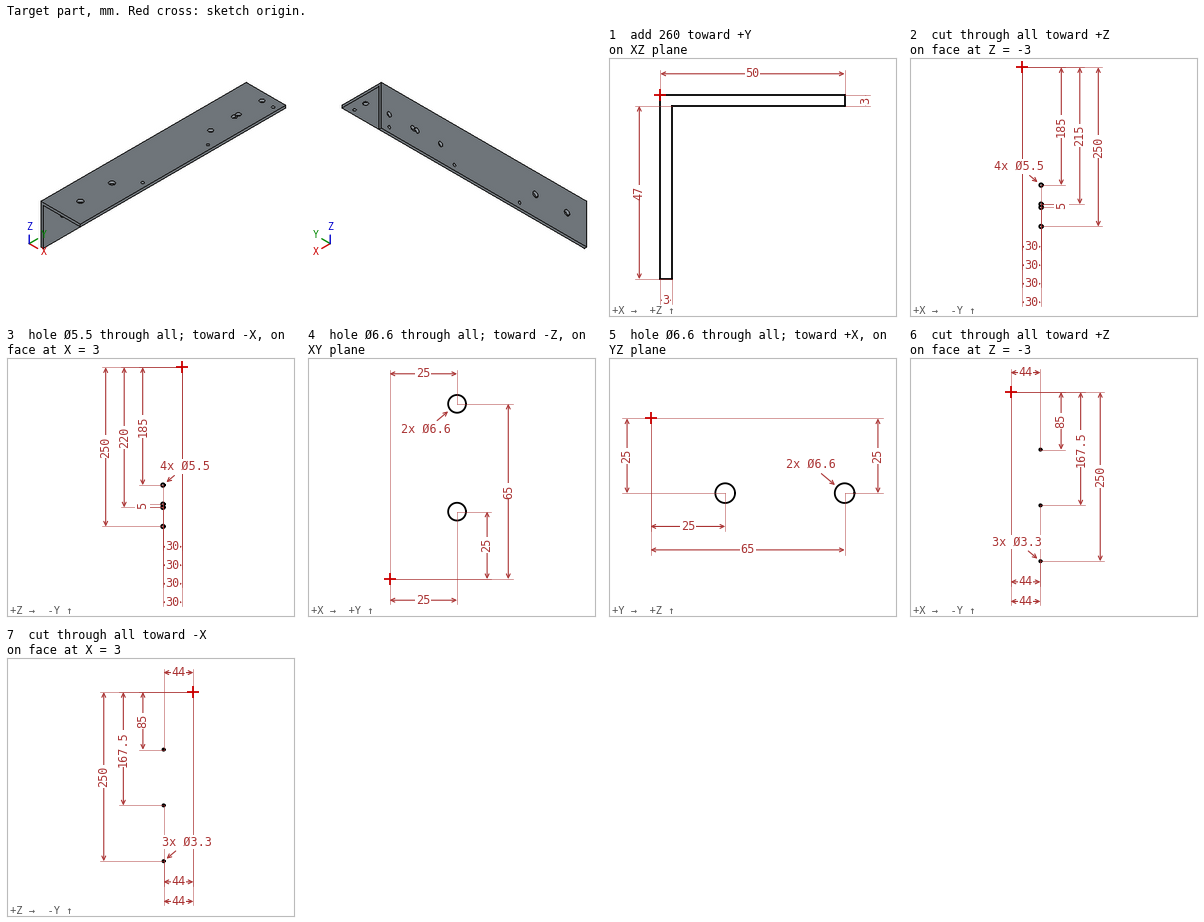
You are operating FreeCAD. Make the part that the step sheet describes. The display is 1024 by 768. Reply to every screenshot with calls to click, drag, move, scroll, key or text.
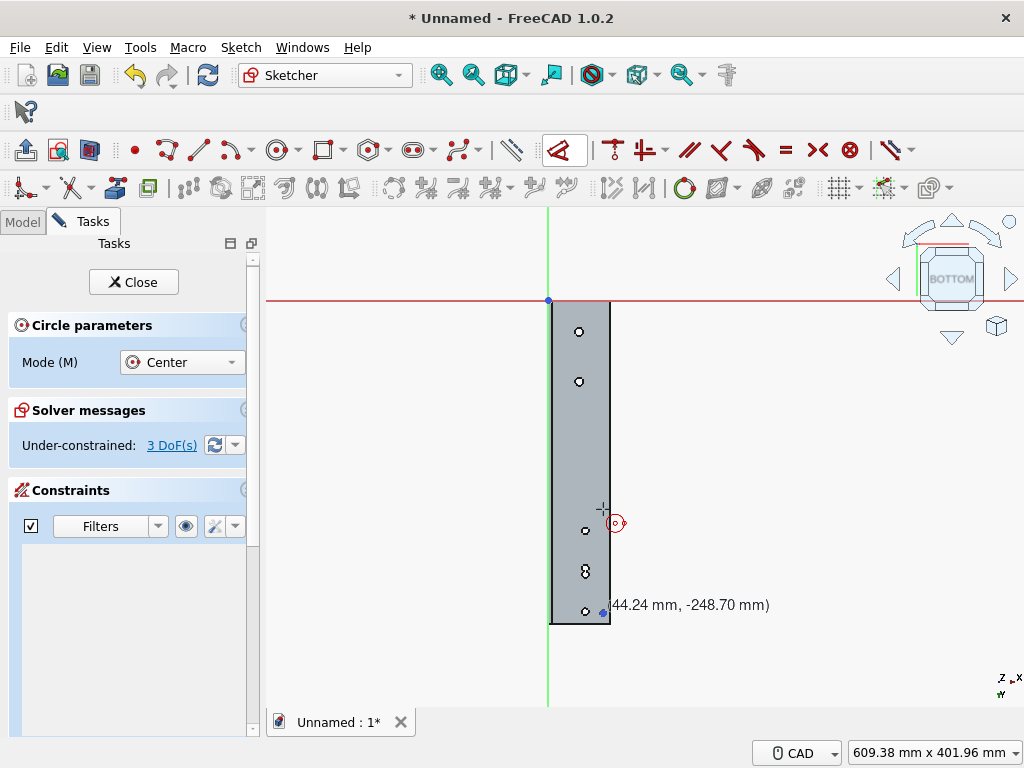
click(603, 509)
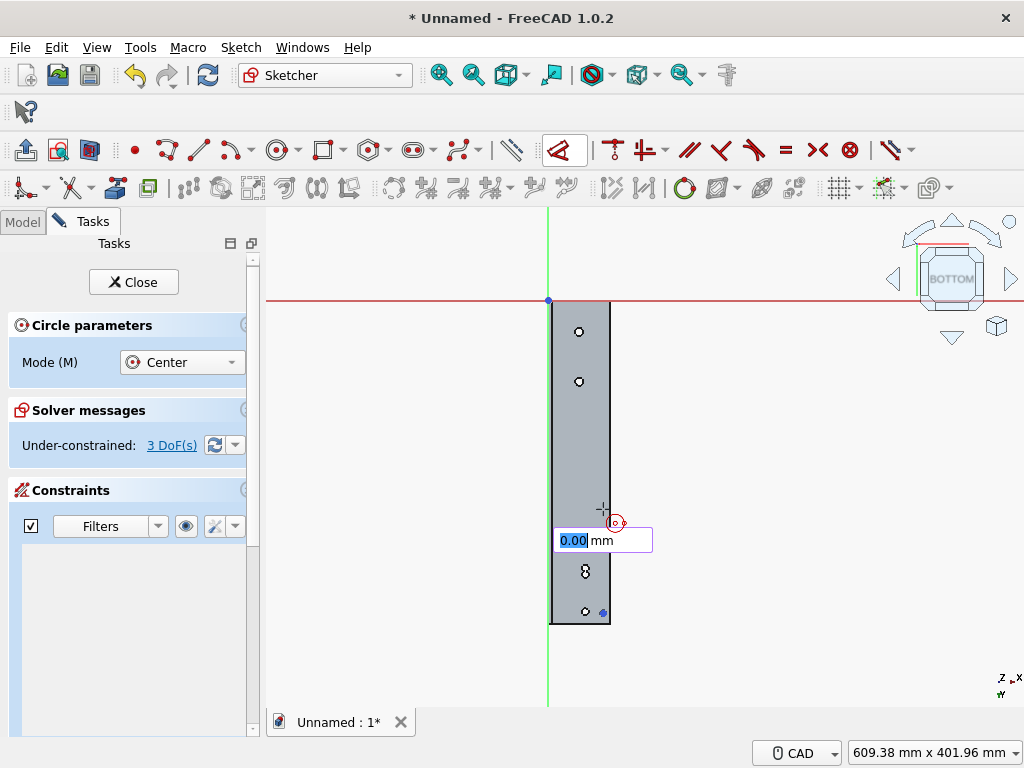
scroll(604, 508, up, 11)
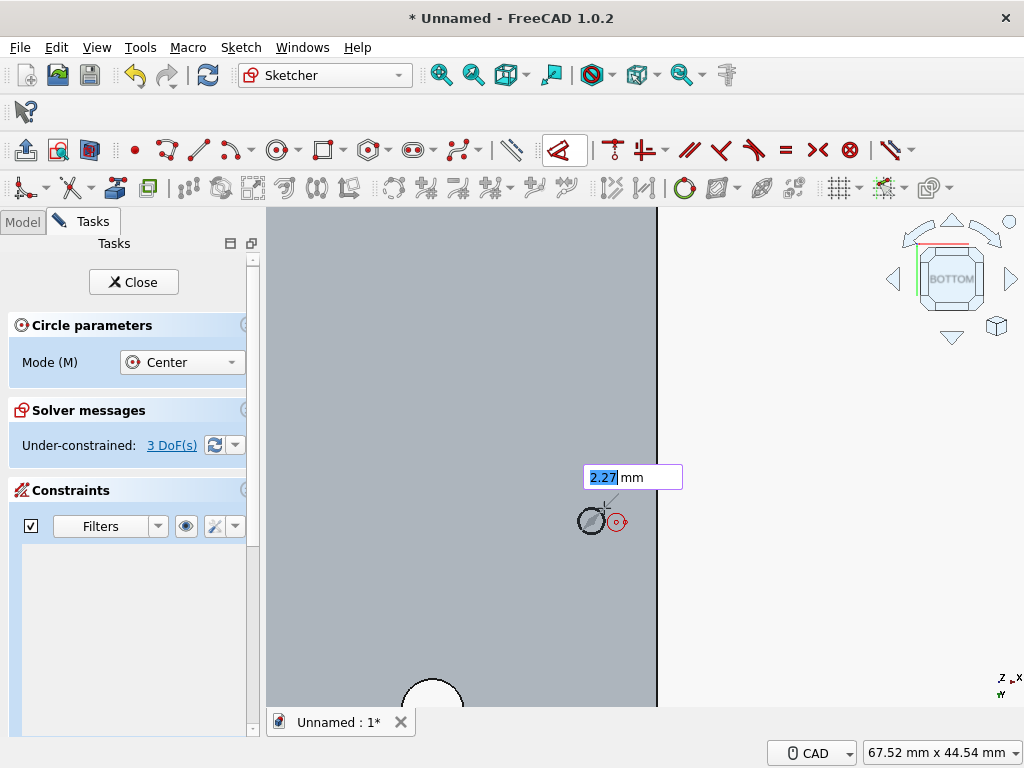
click(603, 500)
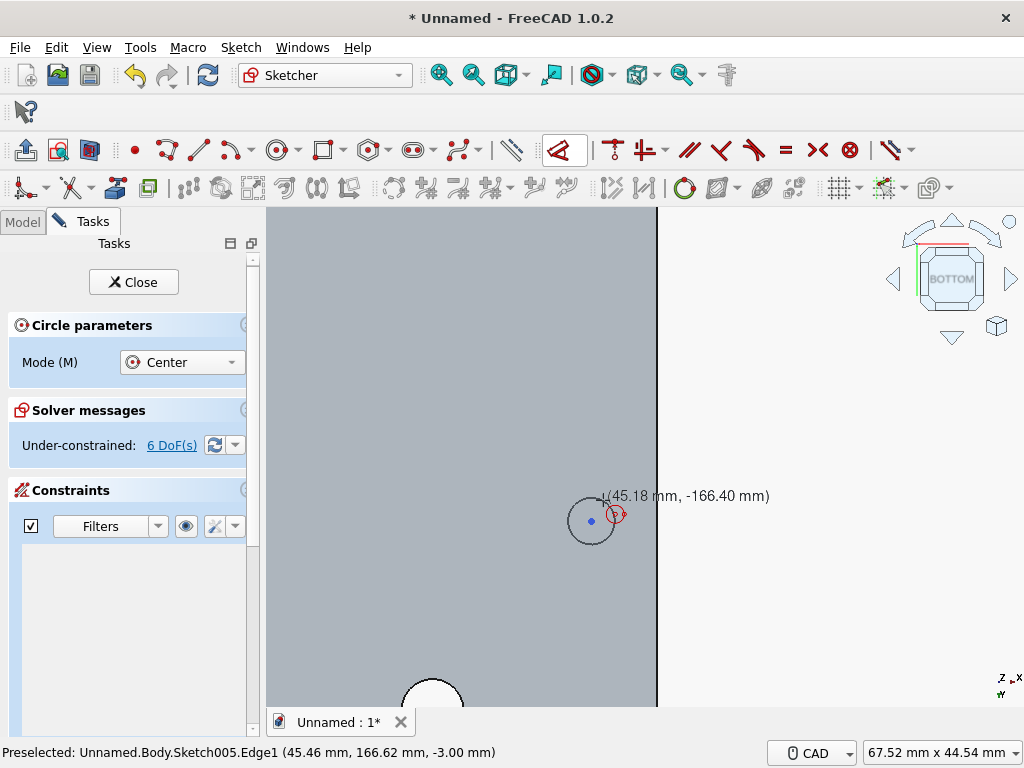
scroll(604, 508, down, 11)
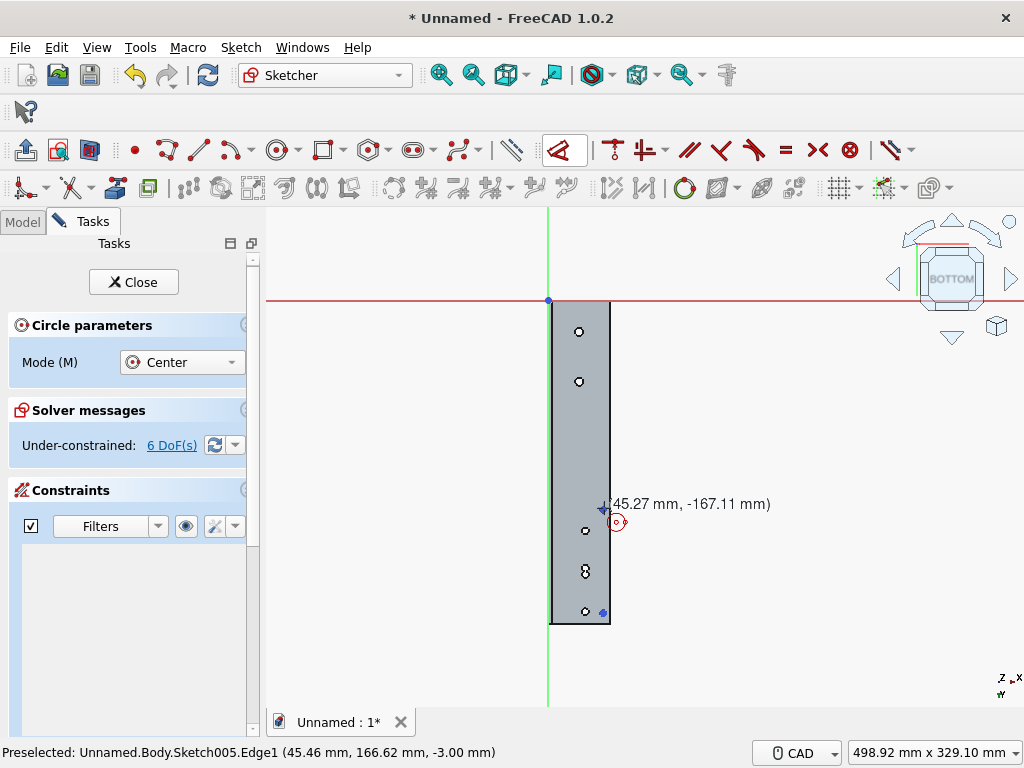
scroll(603, 407, up, 13)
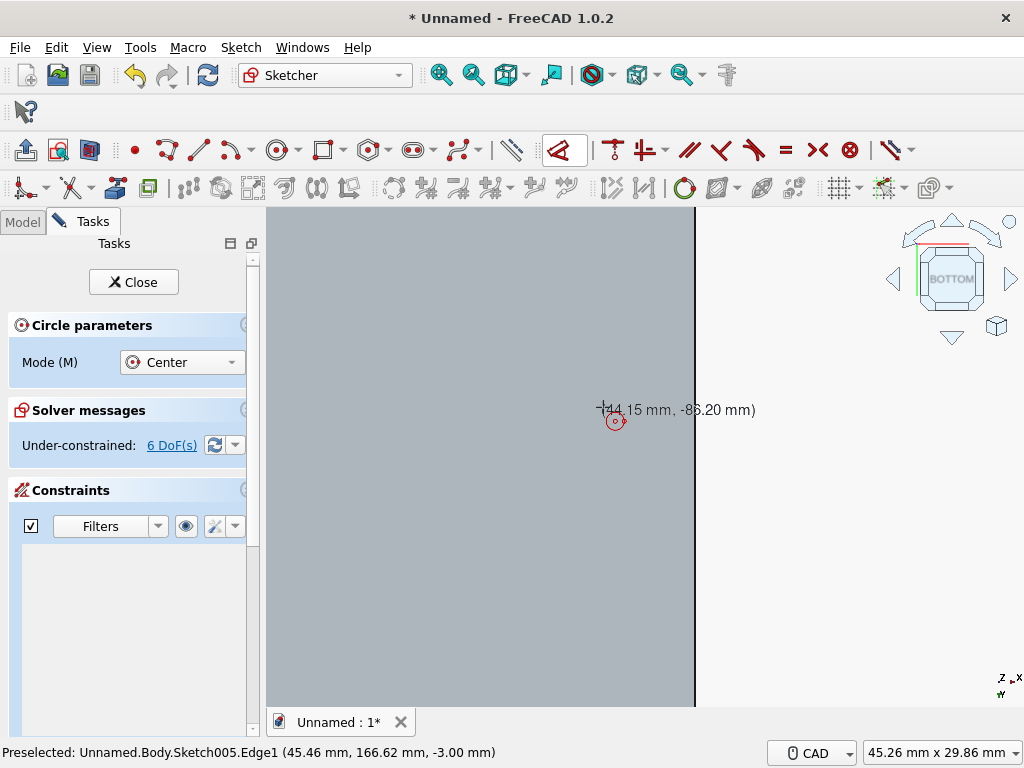
scroll(603, 407, down, 13)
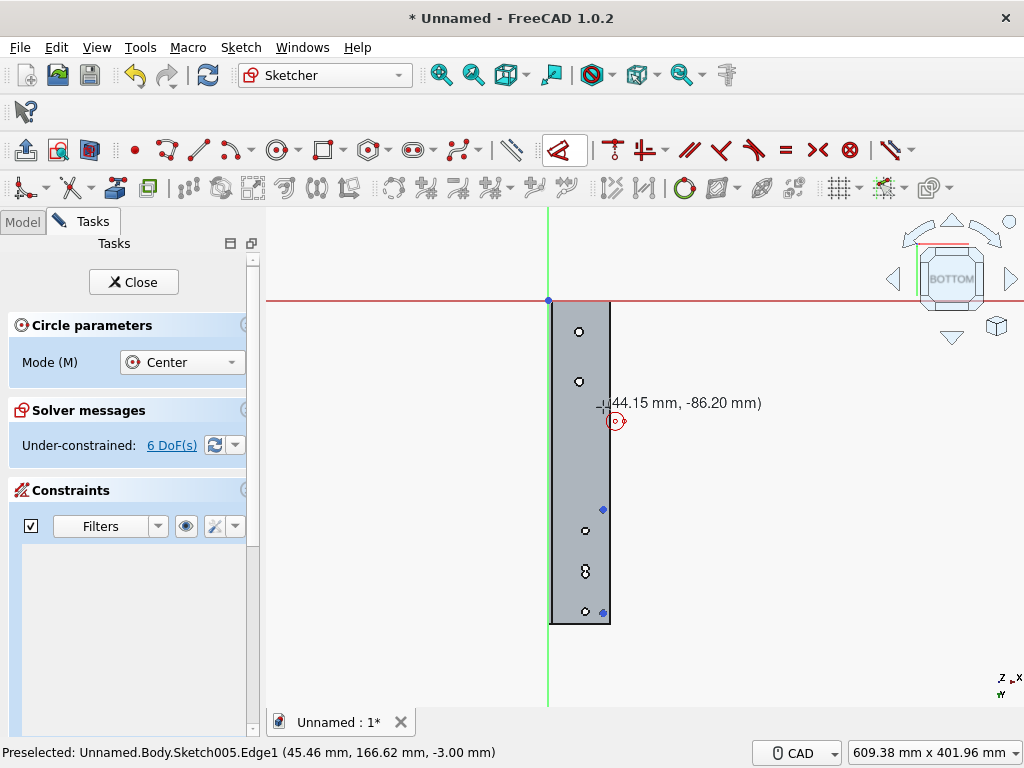
click(603, 407)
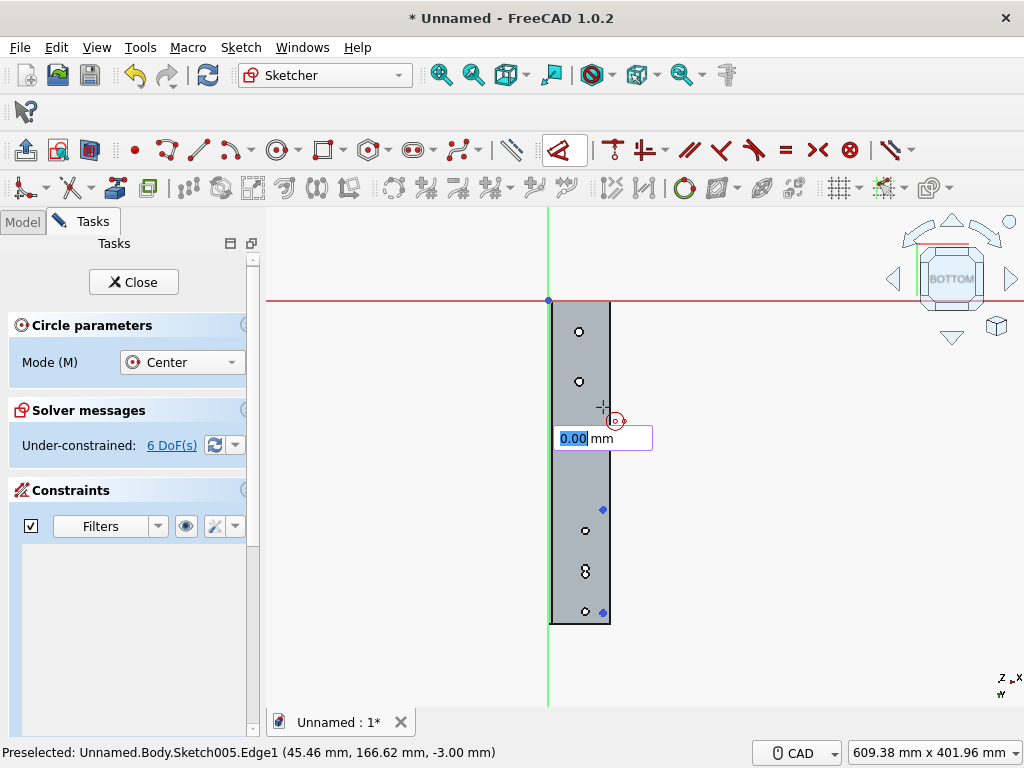
scroll(604, 405, up, 11)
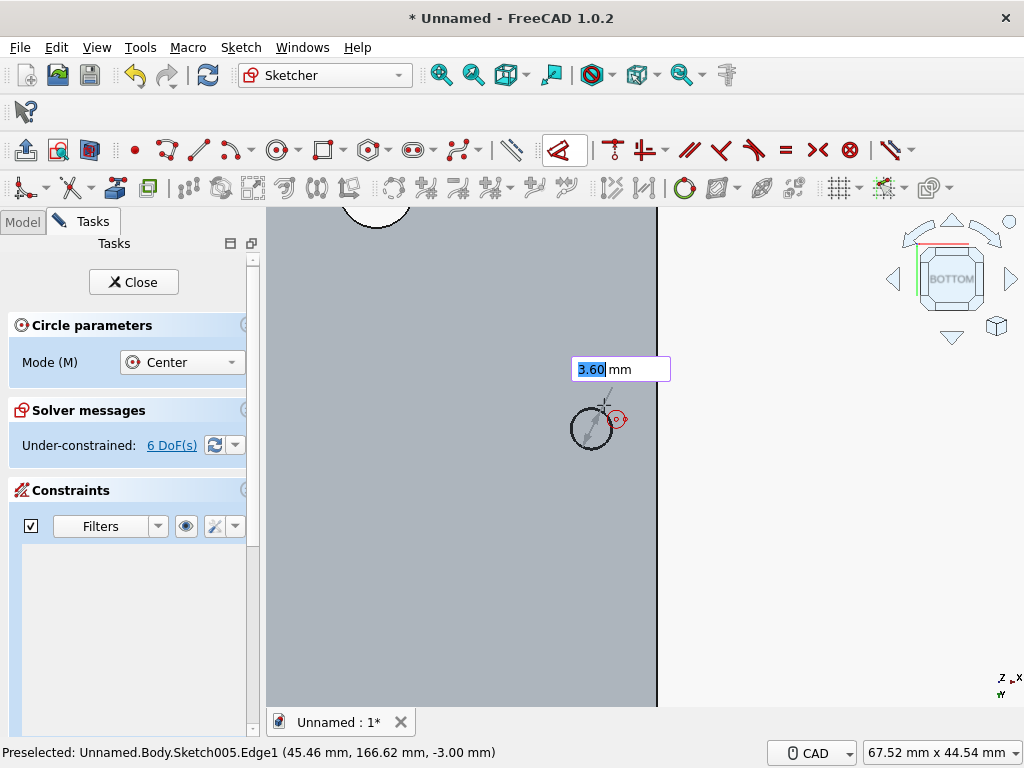
click(603, 402)
key(Escape)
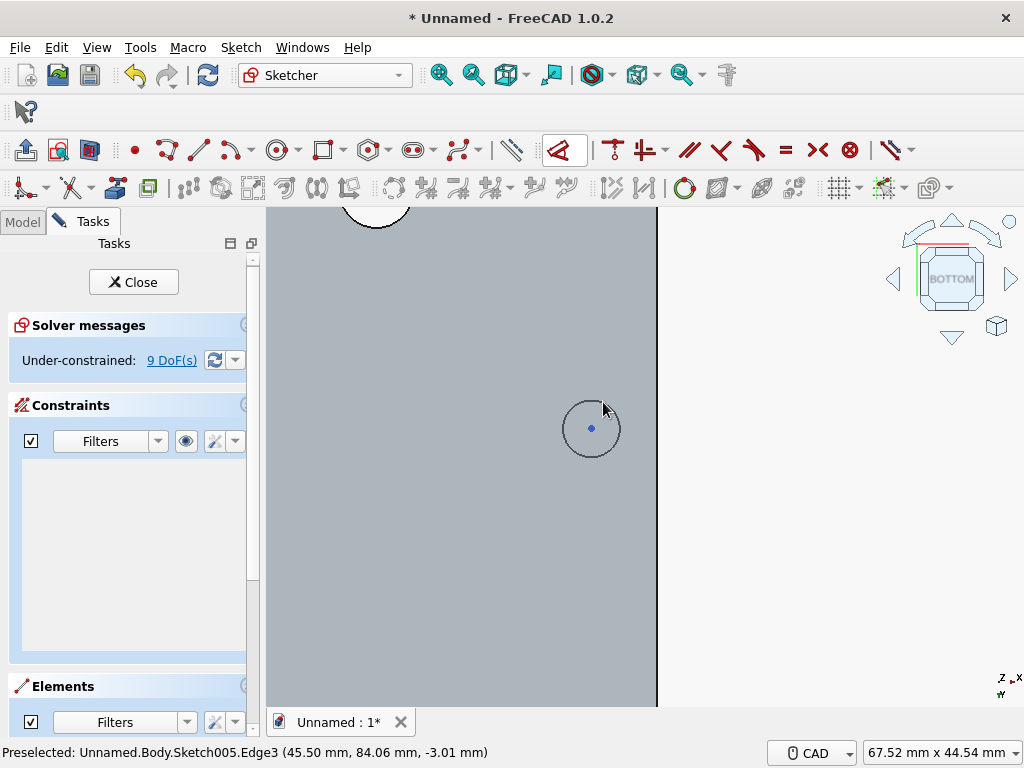
scroll(604, 405, down, 11)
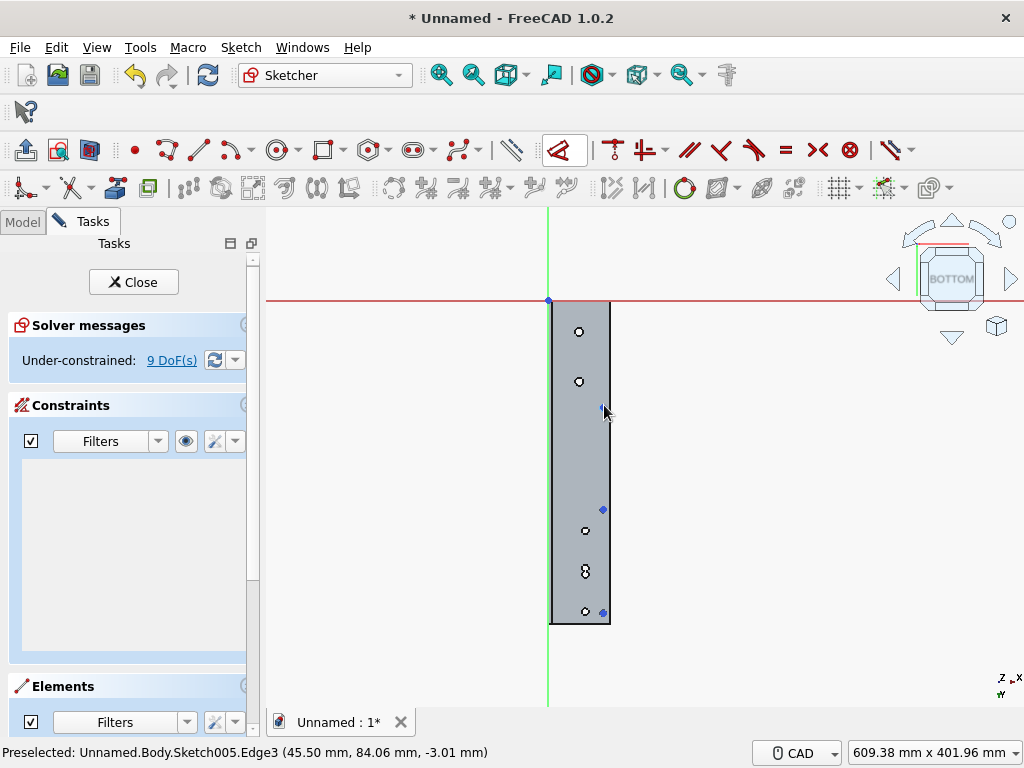
scroll(605, 611, up, 8)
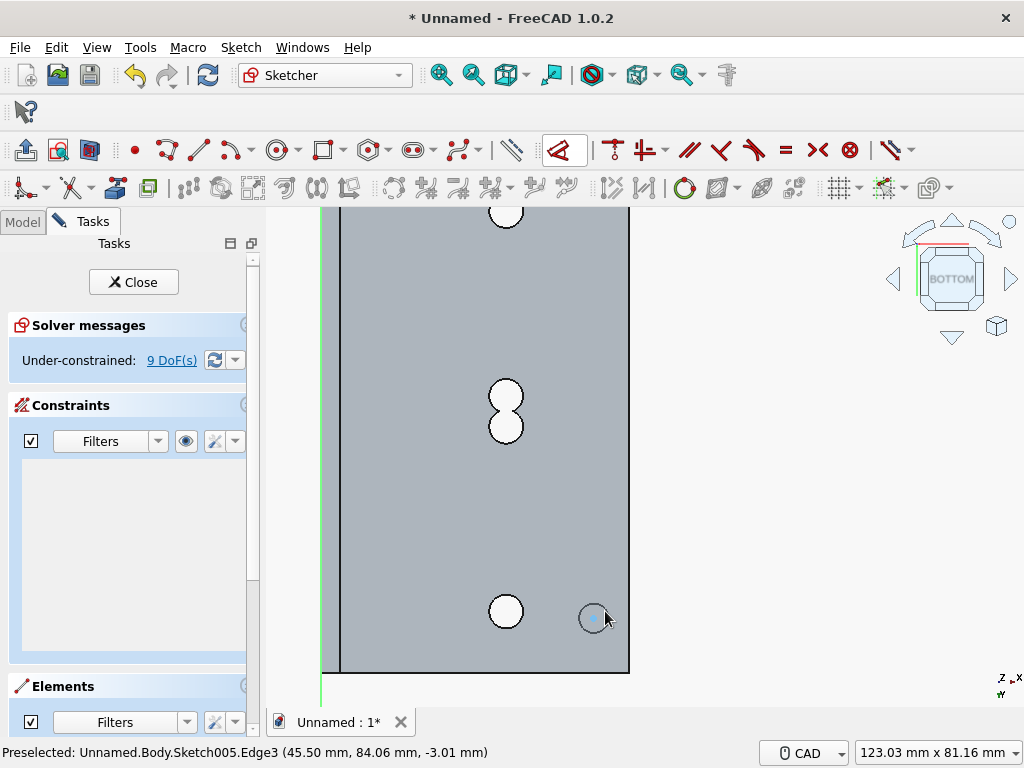
click(604, 608)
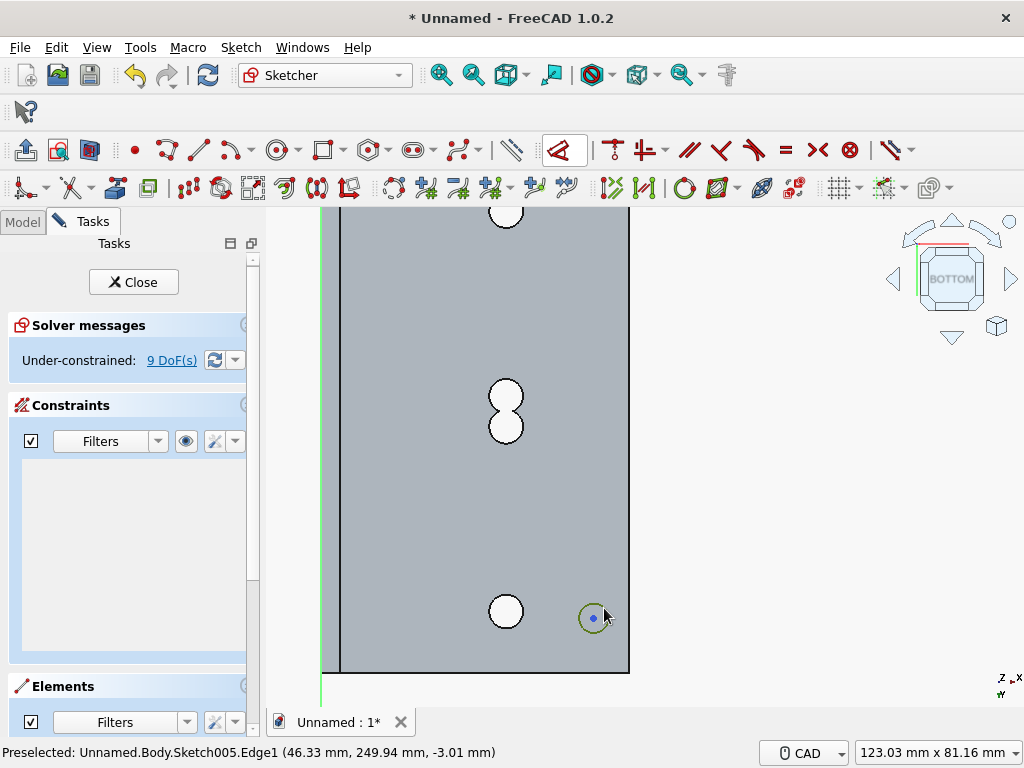
scroll(605, 611, down, 8)